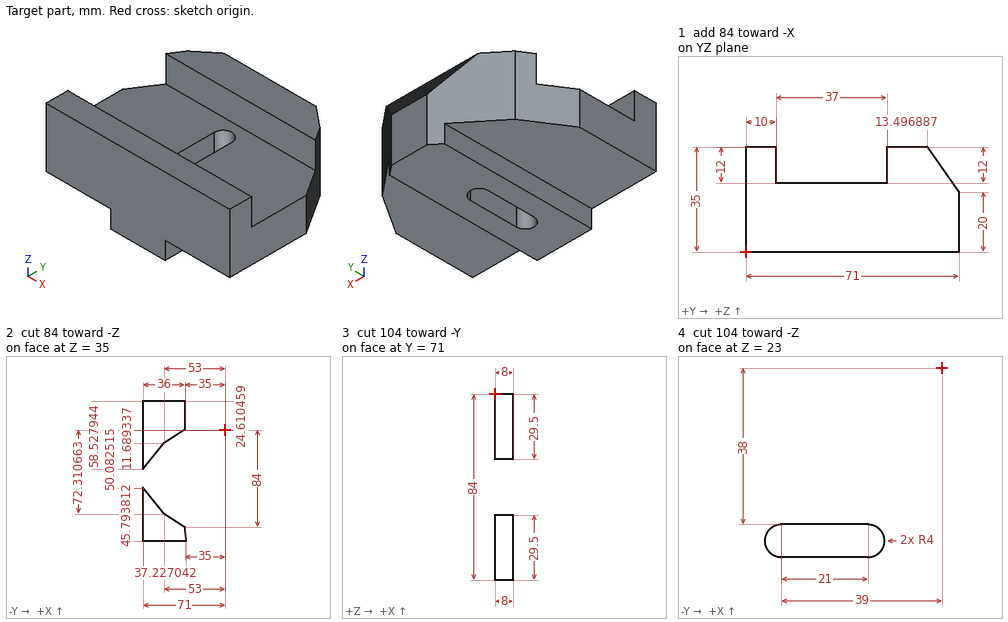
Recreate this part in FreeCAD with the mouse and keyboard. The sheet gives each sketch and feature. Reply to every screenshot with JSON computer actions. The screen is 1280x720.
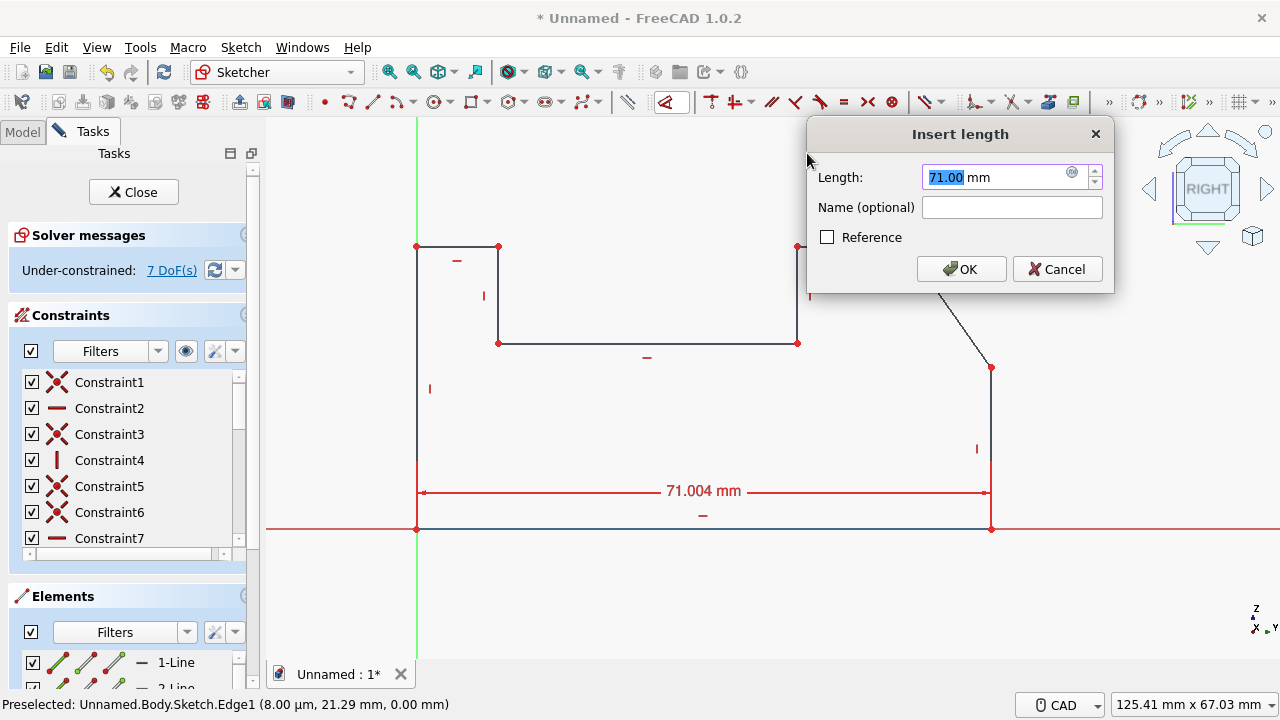
{"action": "type", "text": "71"}
{"action": "key", "text": "Return"}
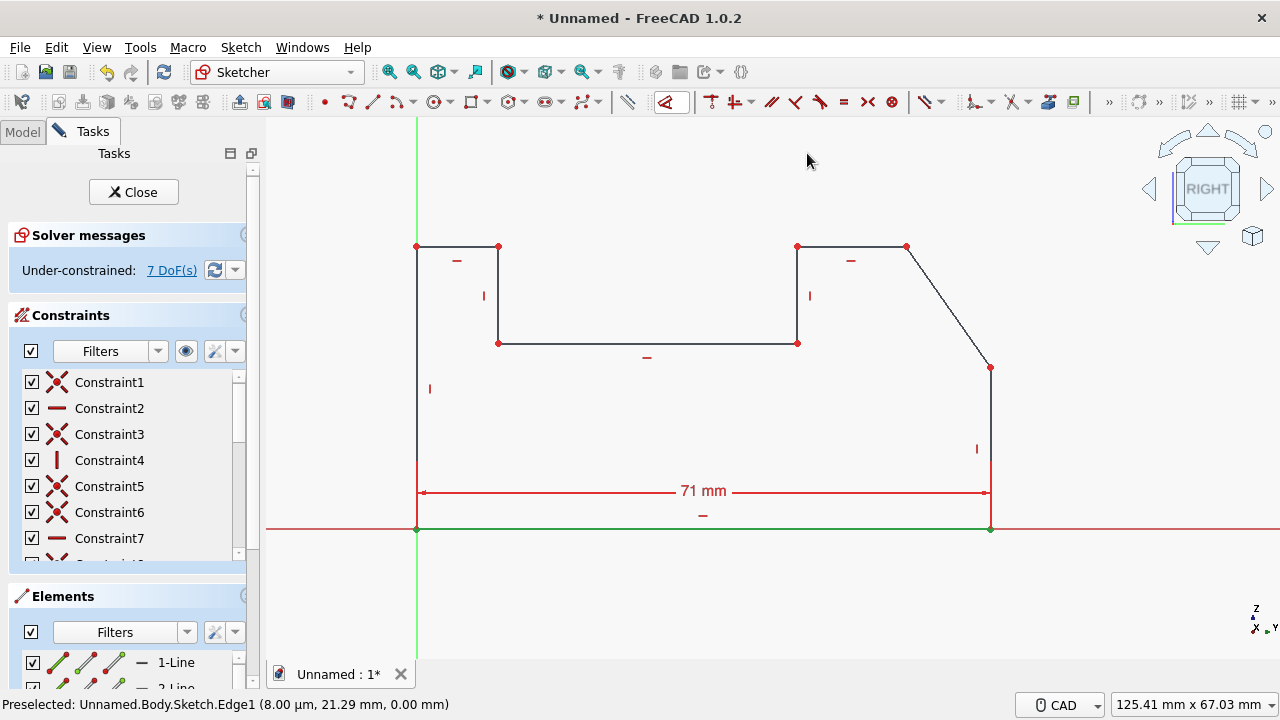
{"action": "left_click", "coordinate": [991, 481]}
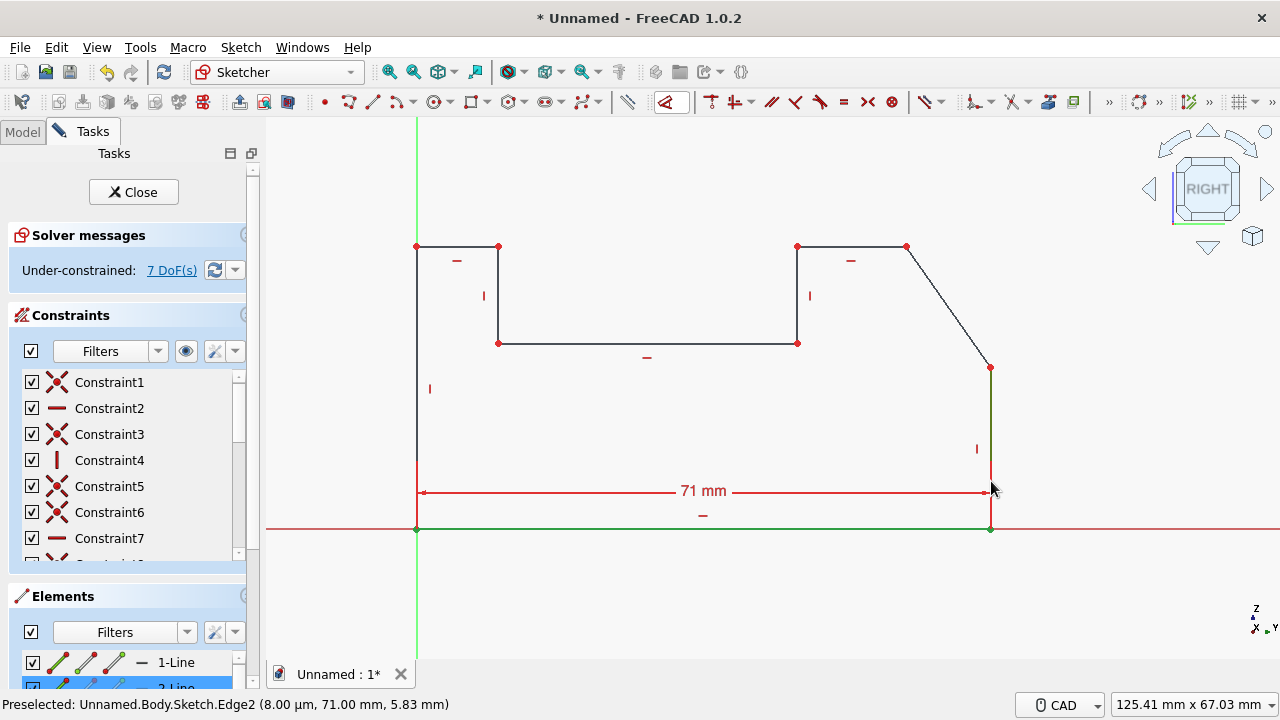
{"action": "left_click", "coordinate": [684, 102]}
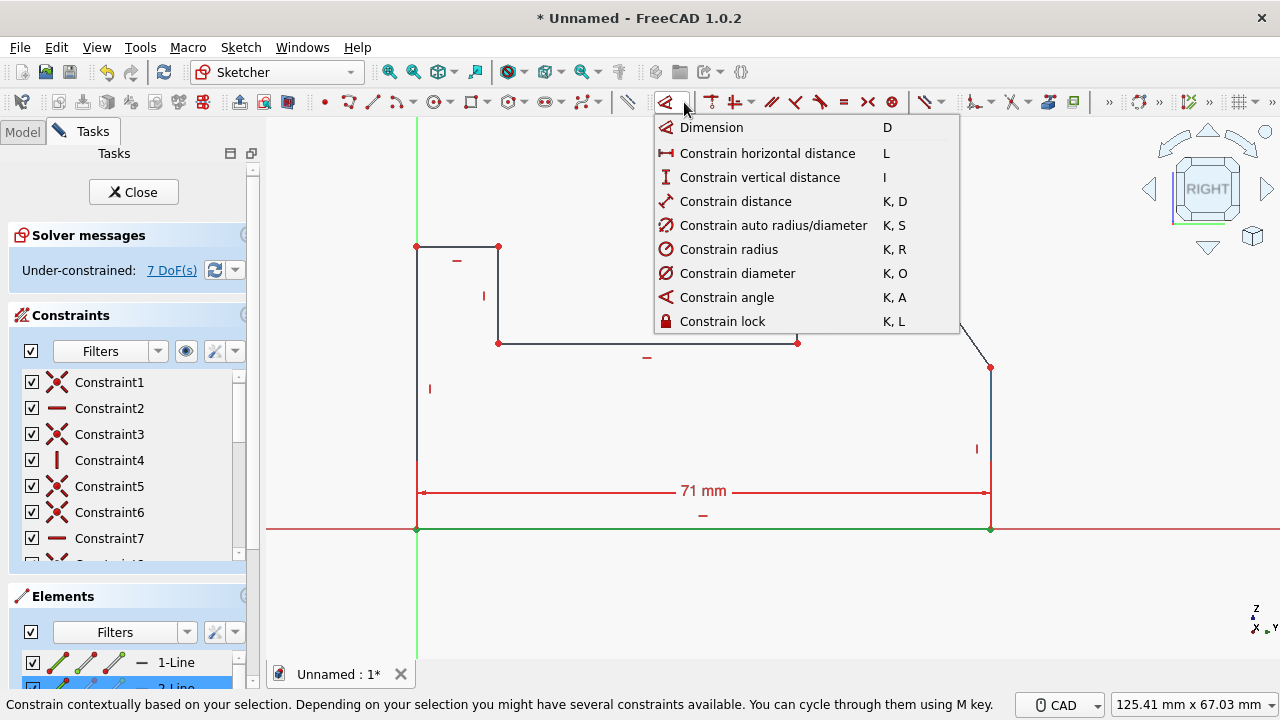
{"action": "left_click", "coordinate": [807, 177]}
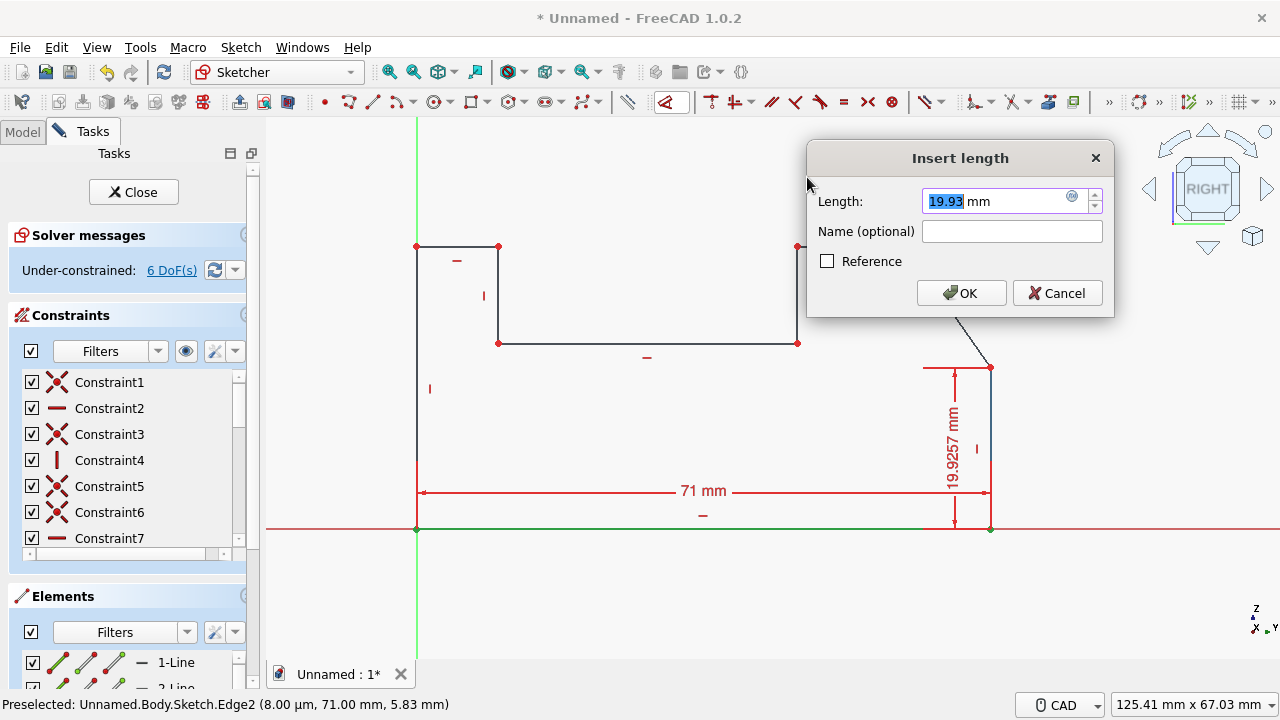
{"action": "type", "text": "20"}
{"action": "key", "text": "Return"}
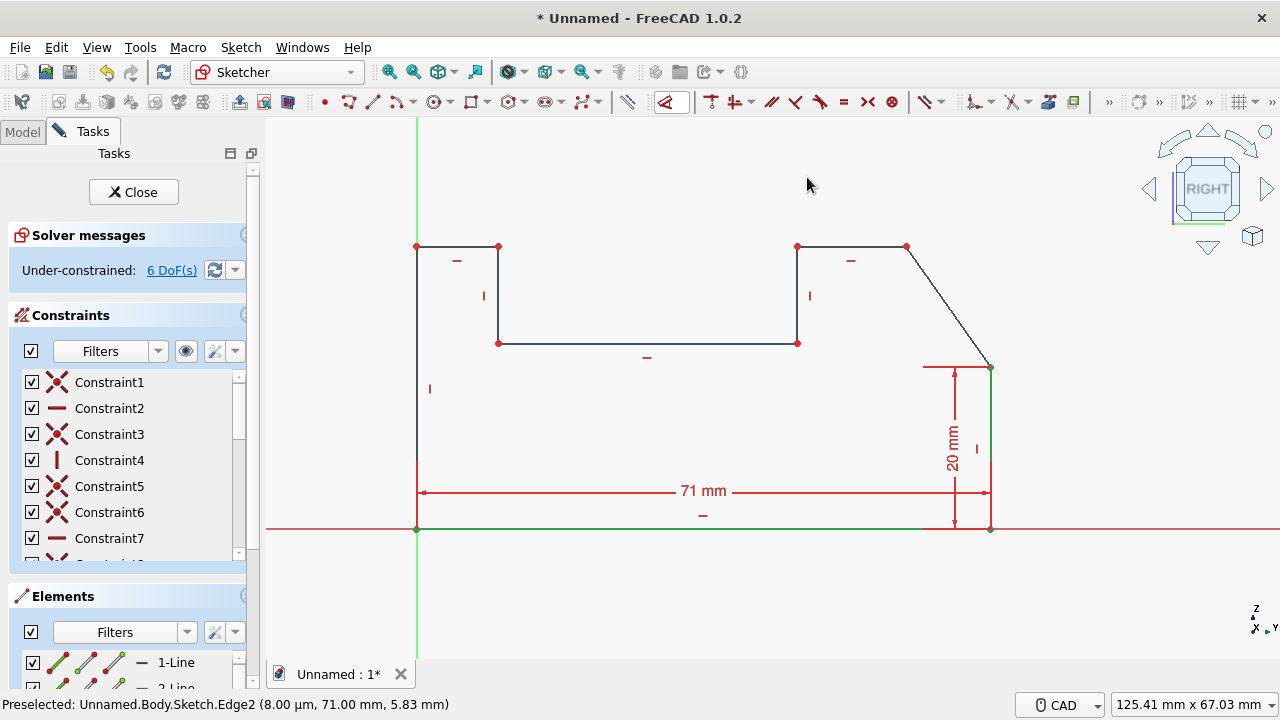
{"action": "left_click", "coordinate": [797, 276]}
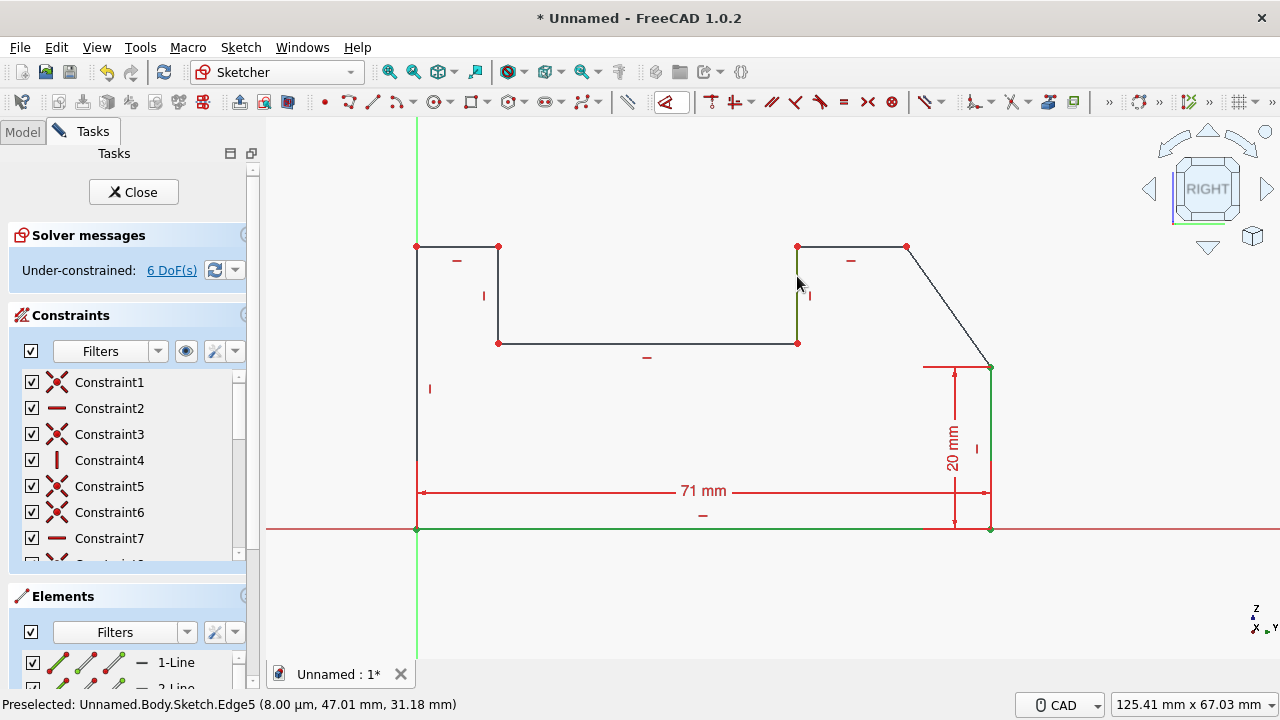
{"action": "key", "text": "i"}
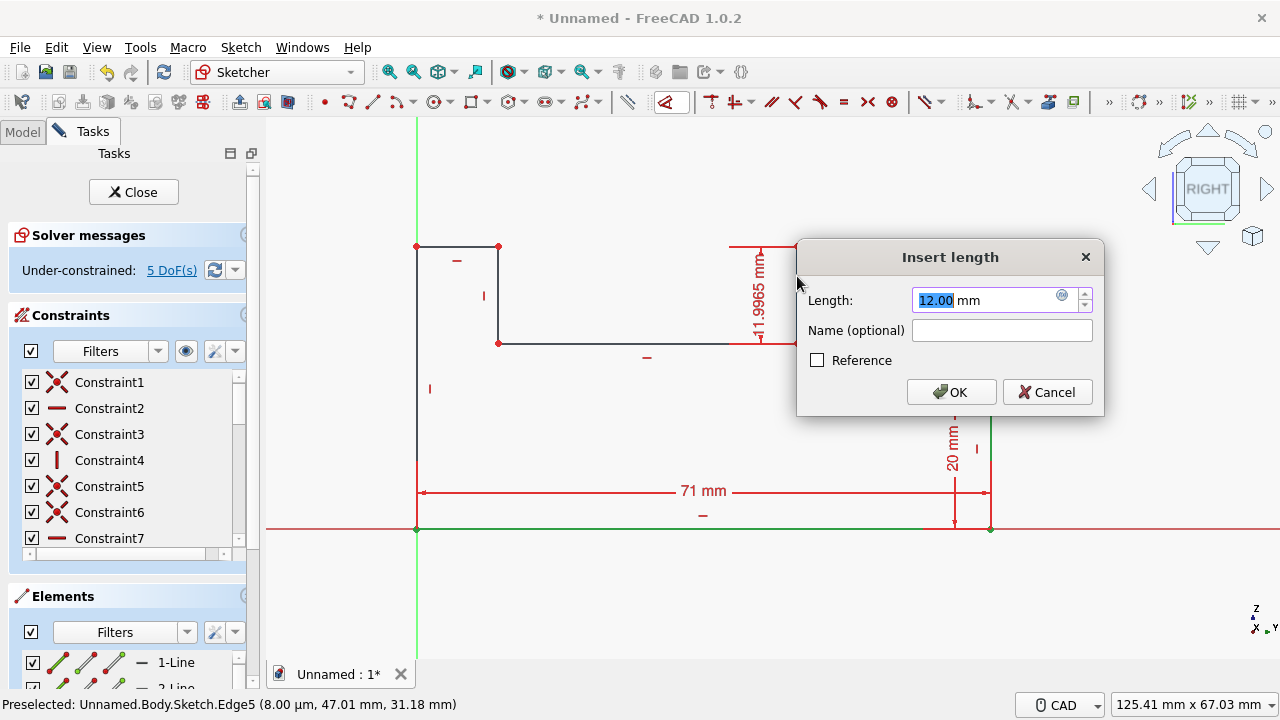
{"action": "type", "text": "12"}
{"action": "key", "text": "Return"}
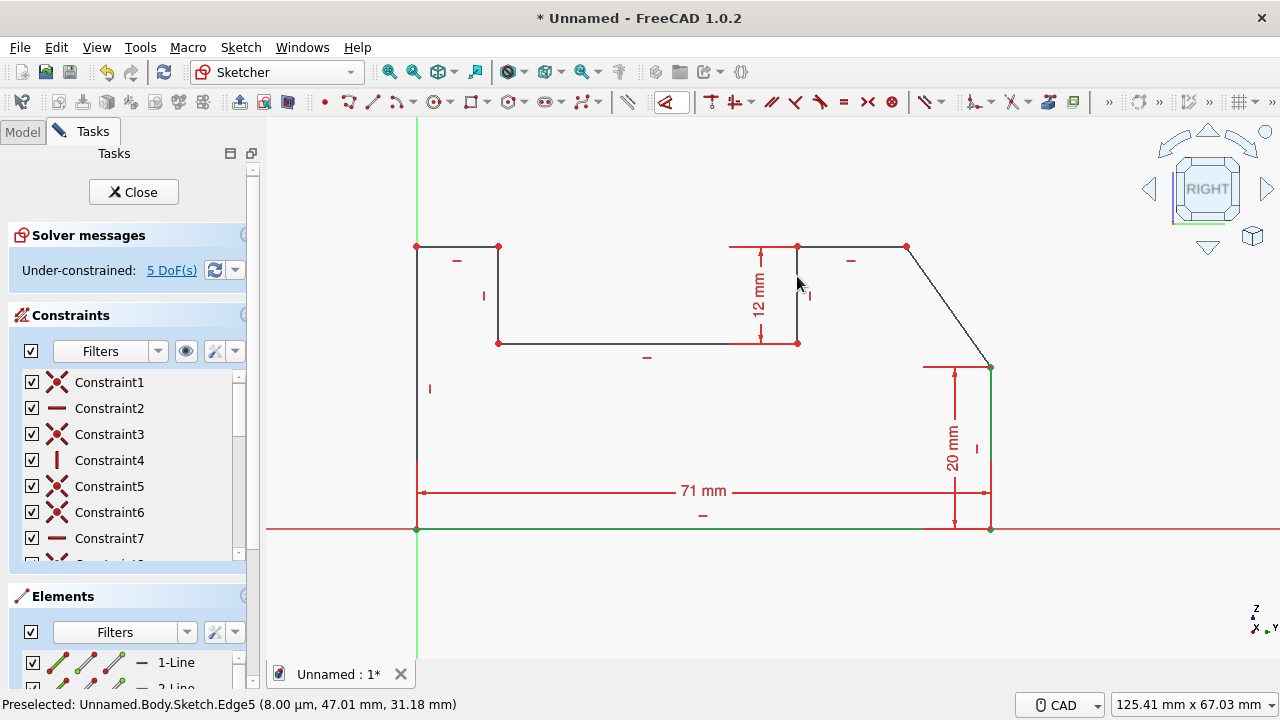
{"action": "left_click", "coordinate": [707, 344]}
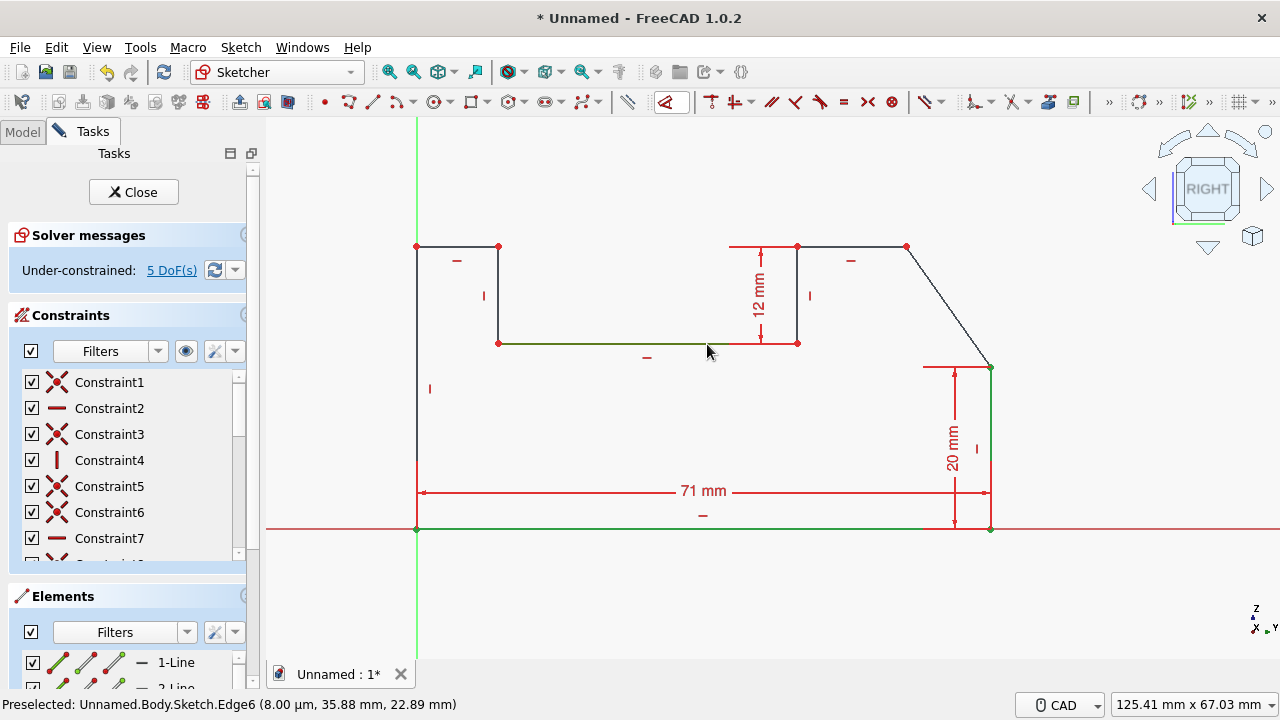
{"action": "left_click", "coordinate": [684, 102]}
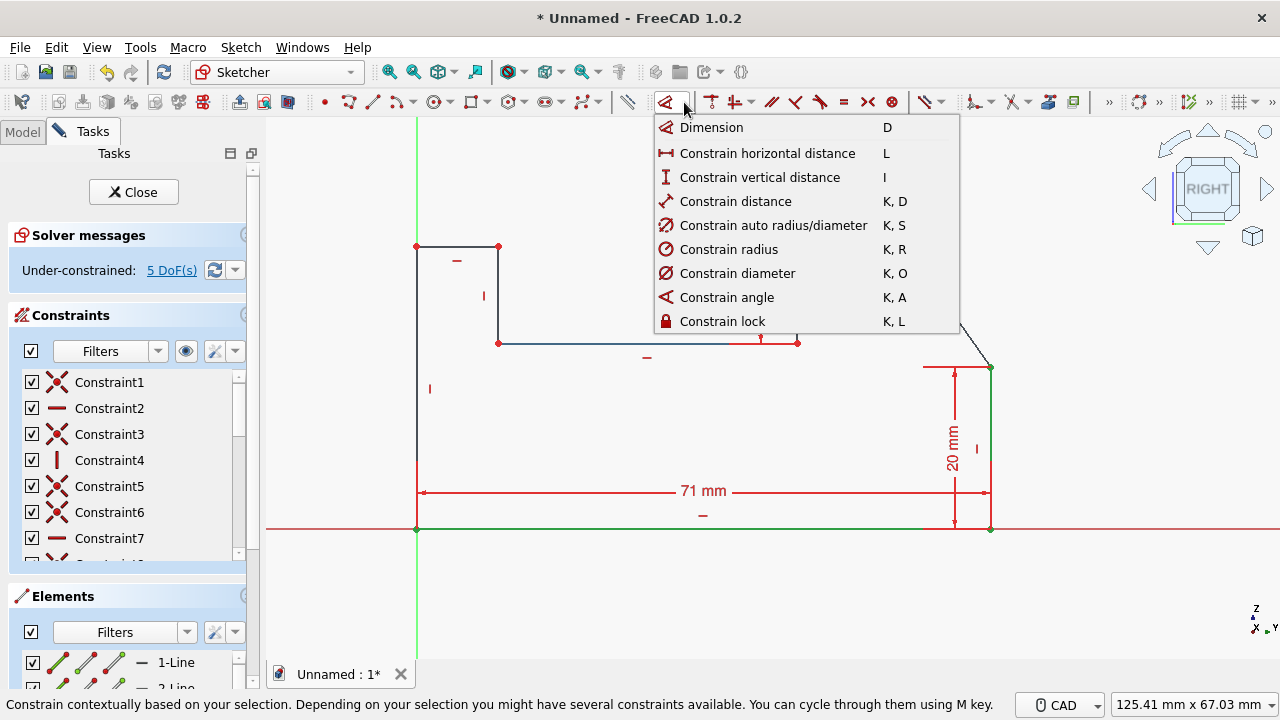
{"action": "left_click", "coordinate": [807, 153]}